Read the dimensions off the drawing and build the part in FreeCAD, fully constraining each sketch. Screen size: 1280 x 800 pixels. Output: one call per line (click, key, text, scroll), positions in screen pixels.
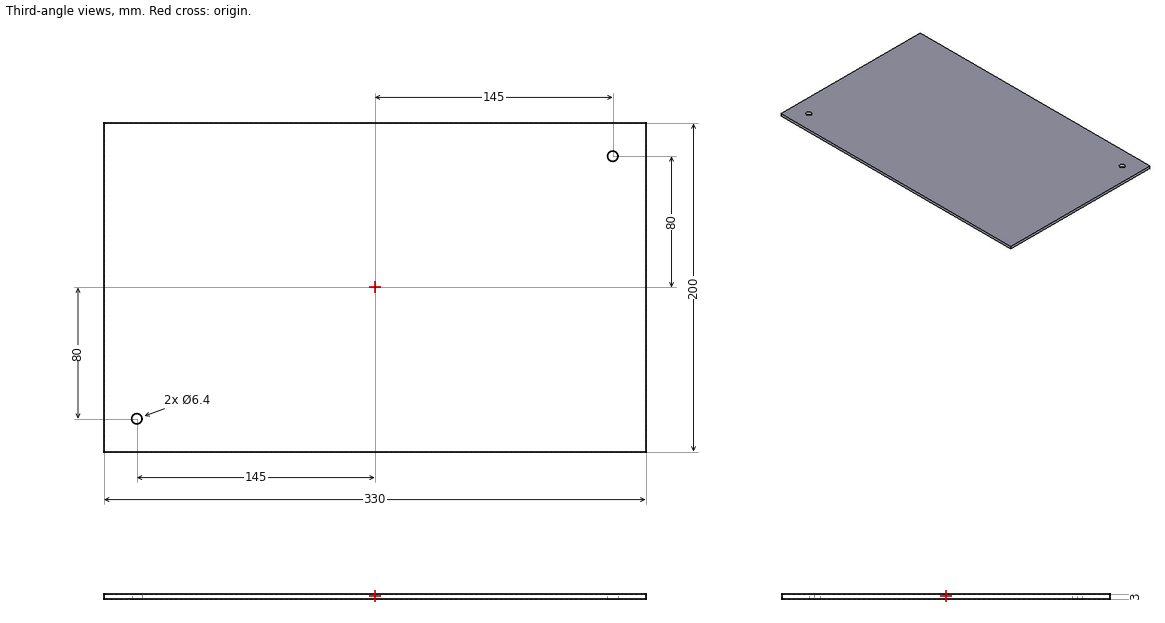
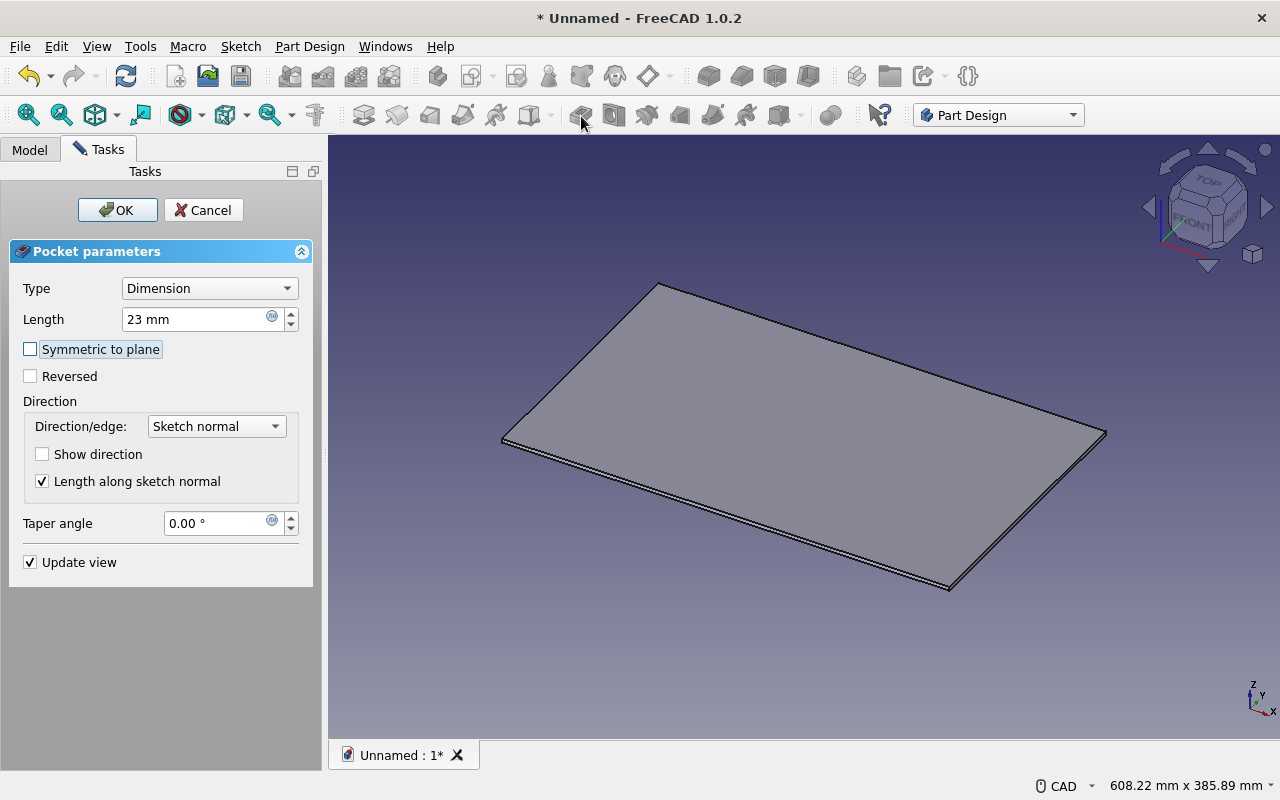
click(31, 349)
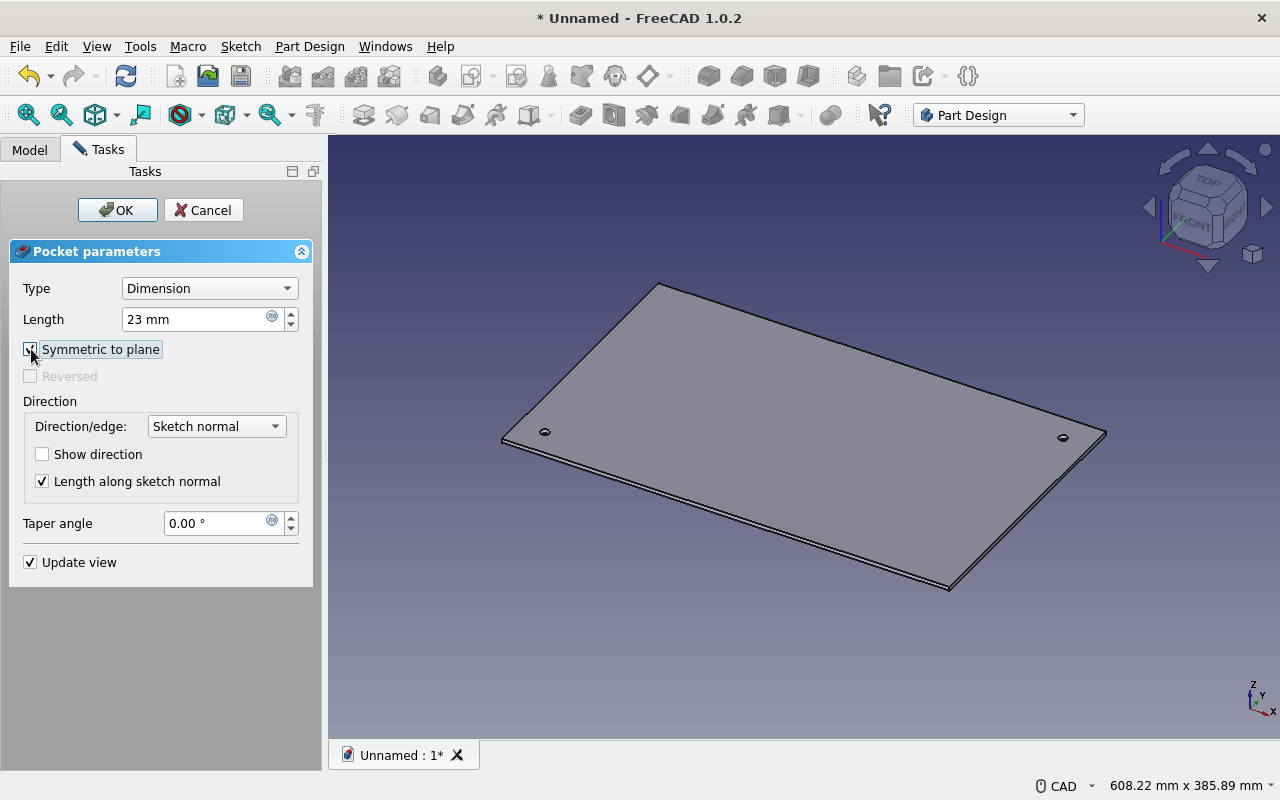
click(118, 210)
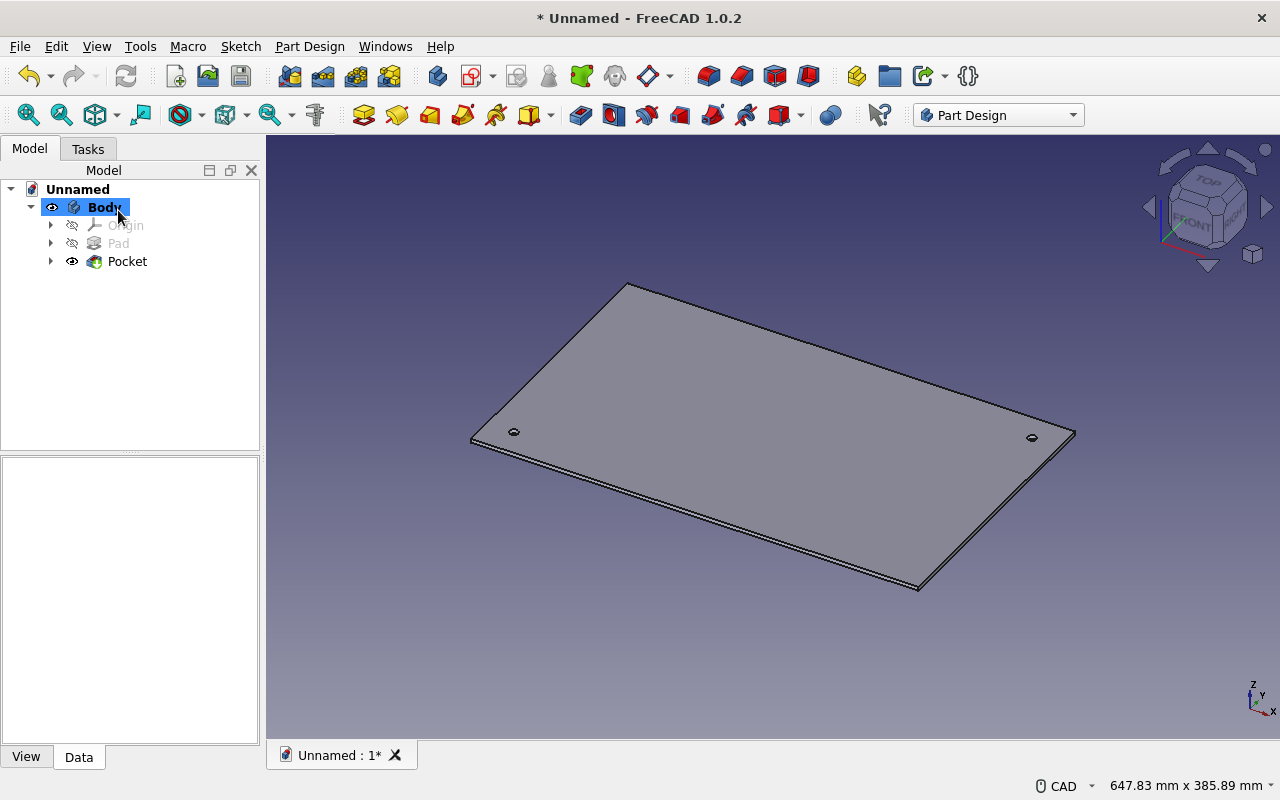
key(0)